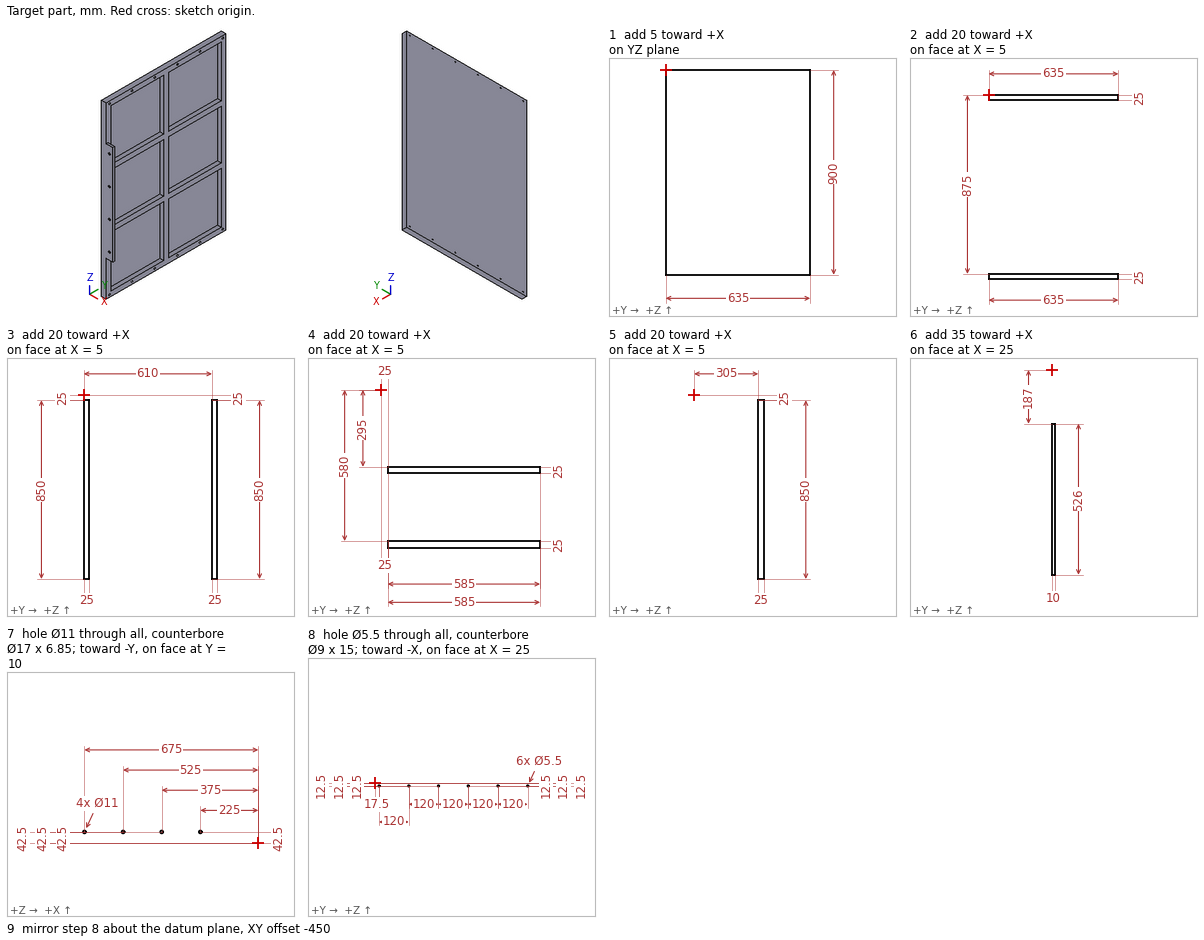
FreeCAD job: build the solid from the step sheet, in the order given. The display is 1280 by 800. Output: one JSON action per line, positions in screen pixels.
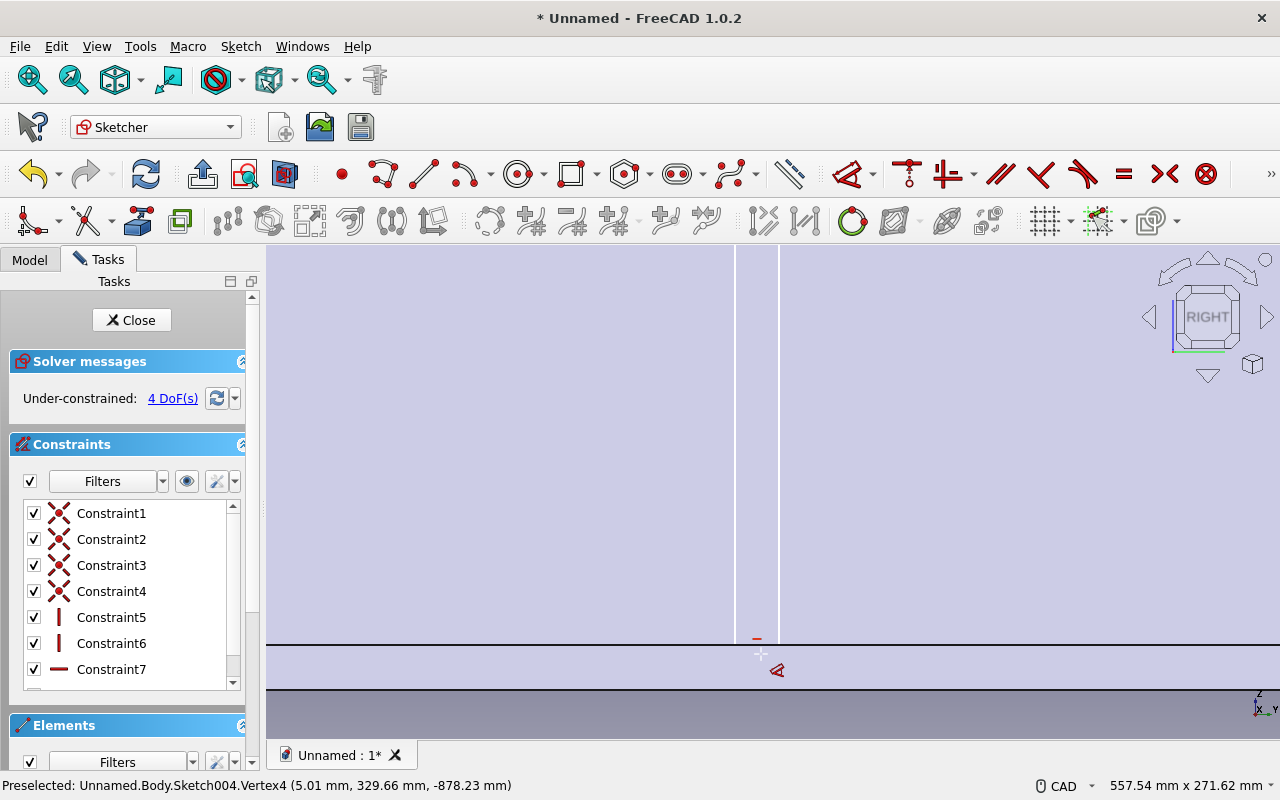
{"action": "left_click", "coordinate": [757, 651]}
{"action": "left_click", "coordinate": [757, 685]}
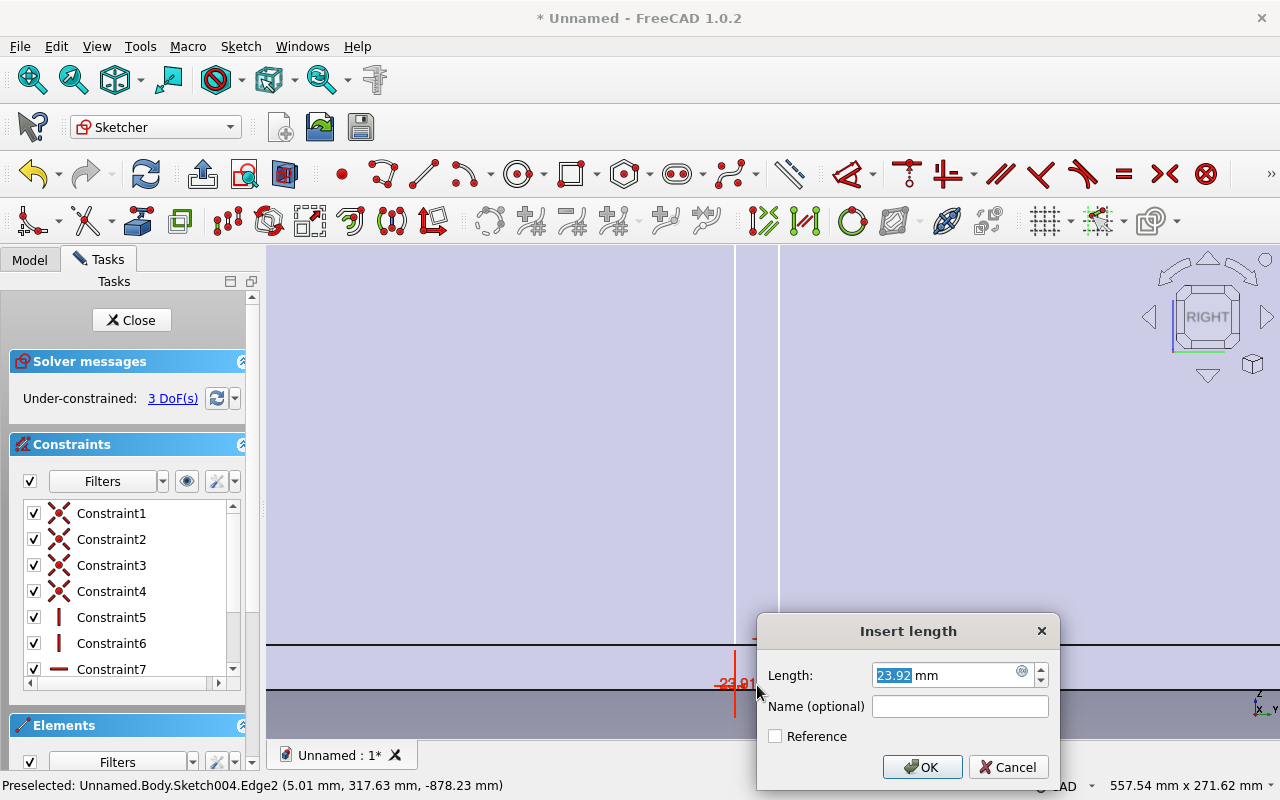
{"action": "type", "text": "25"}
{"action": "key", "text": "Return"}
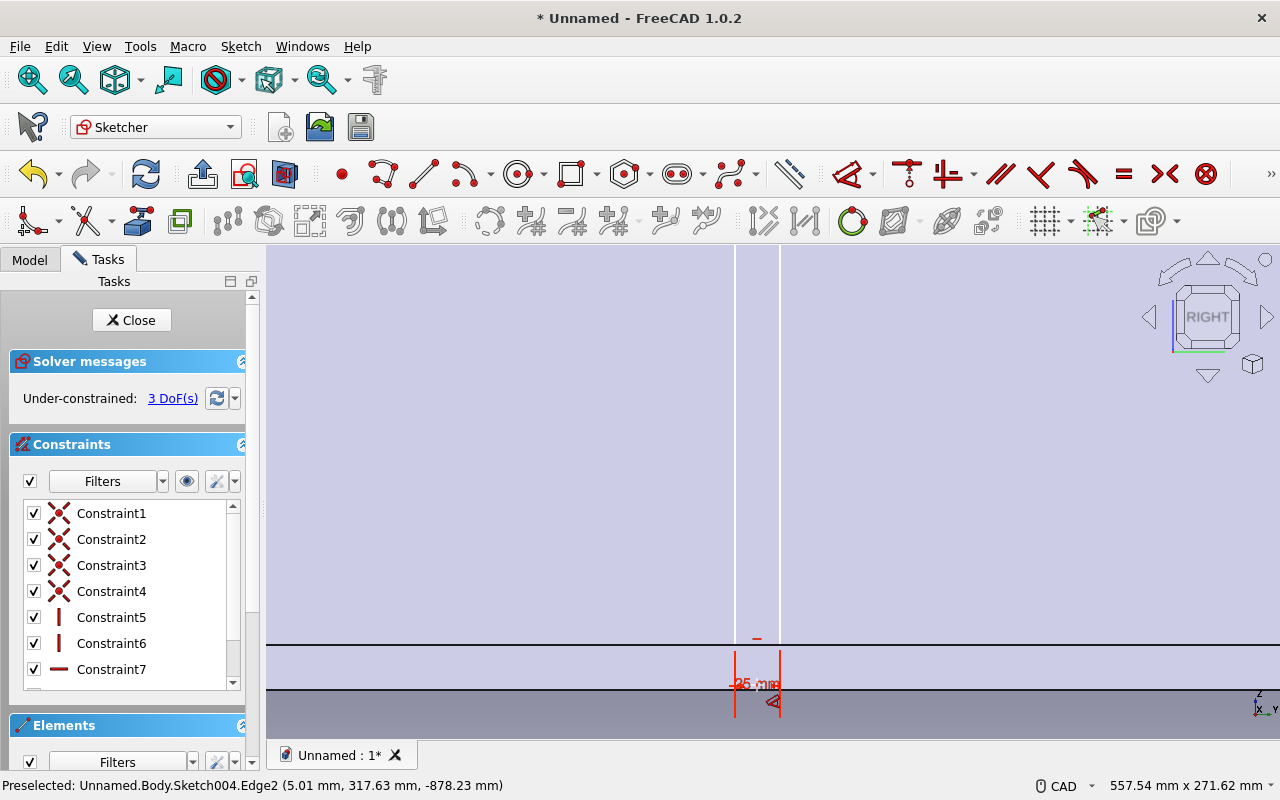
{"action": "scroll", "coordinate": [761, 655], "scroll_direction": "down", "scroll_amount": 8}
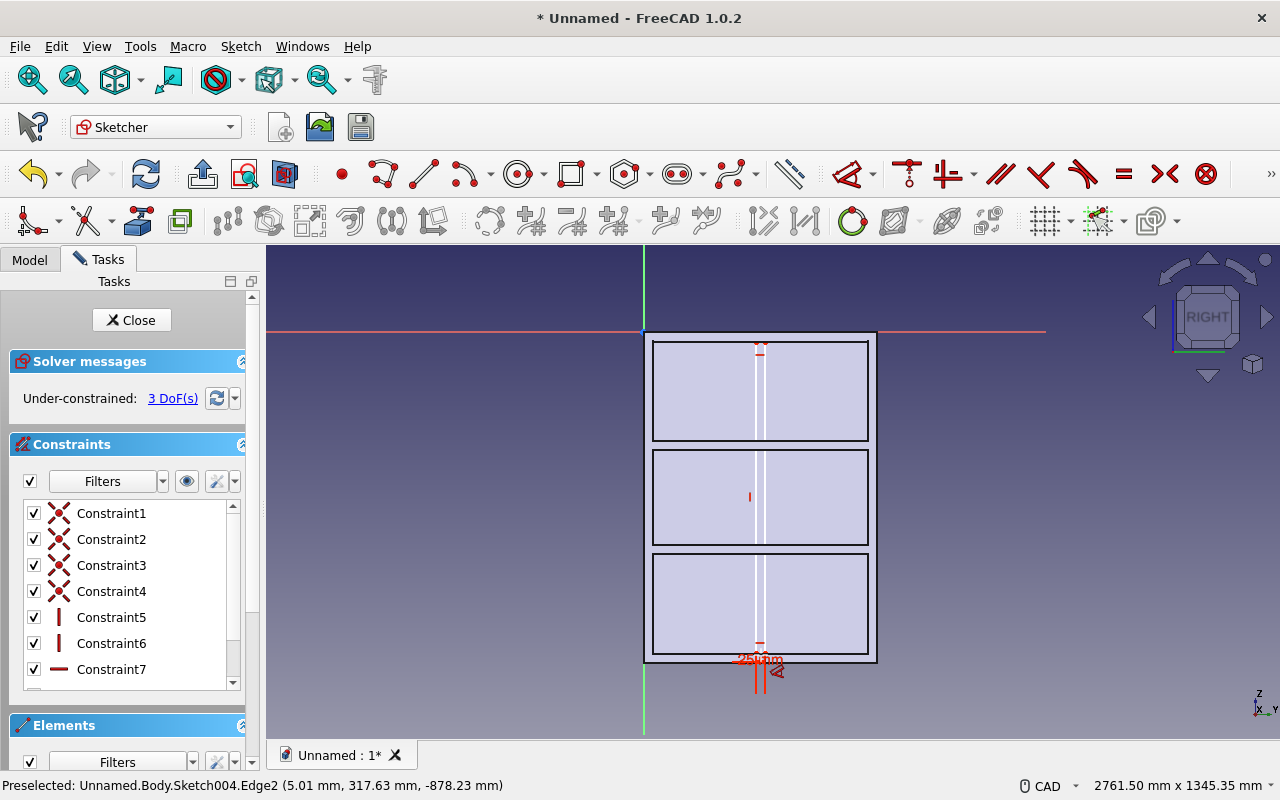
{"action": "scroll", "coordinate": [756, 592], "scroll_direction": "up", "scroll_amount": 3}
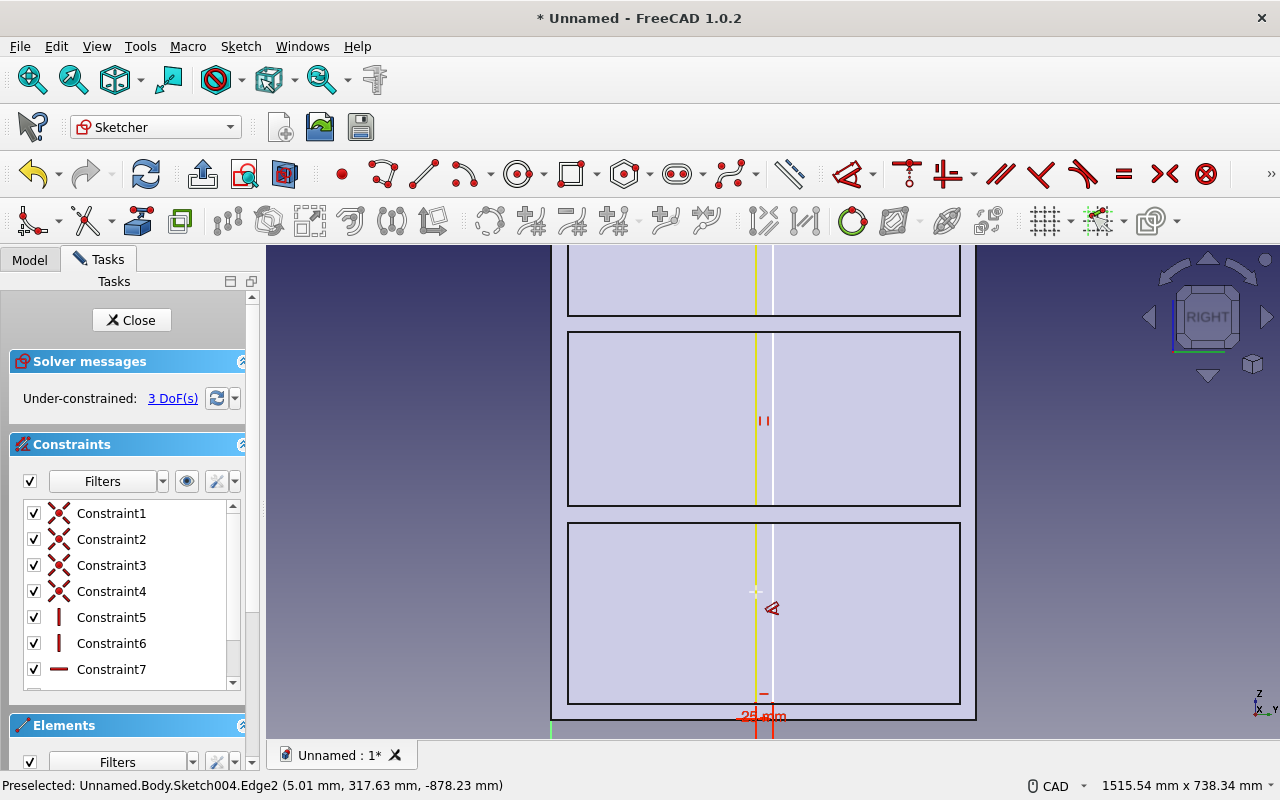
{"action": "left_click", "coordinate": [756, 592]}
{"action": "left_click", "coordinate": [790, 489]}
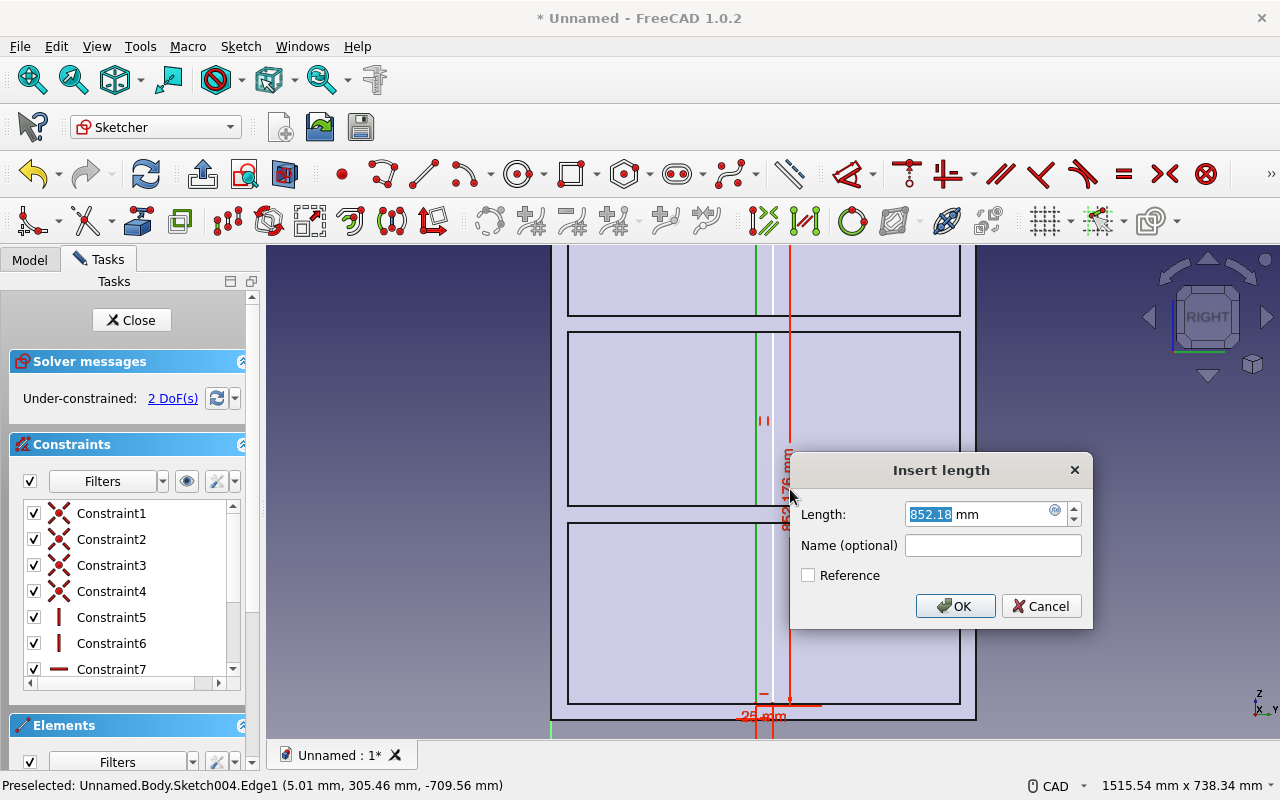
{"action": "type", "text": "850"}
{"action": "key", "text": "Return"}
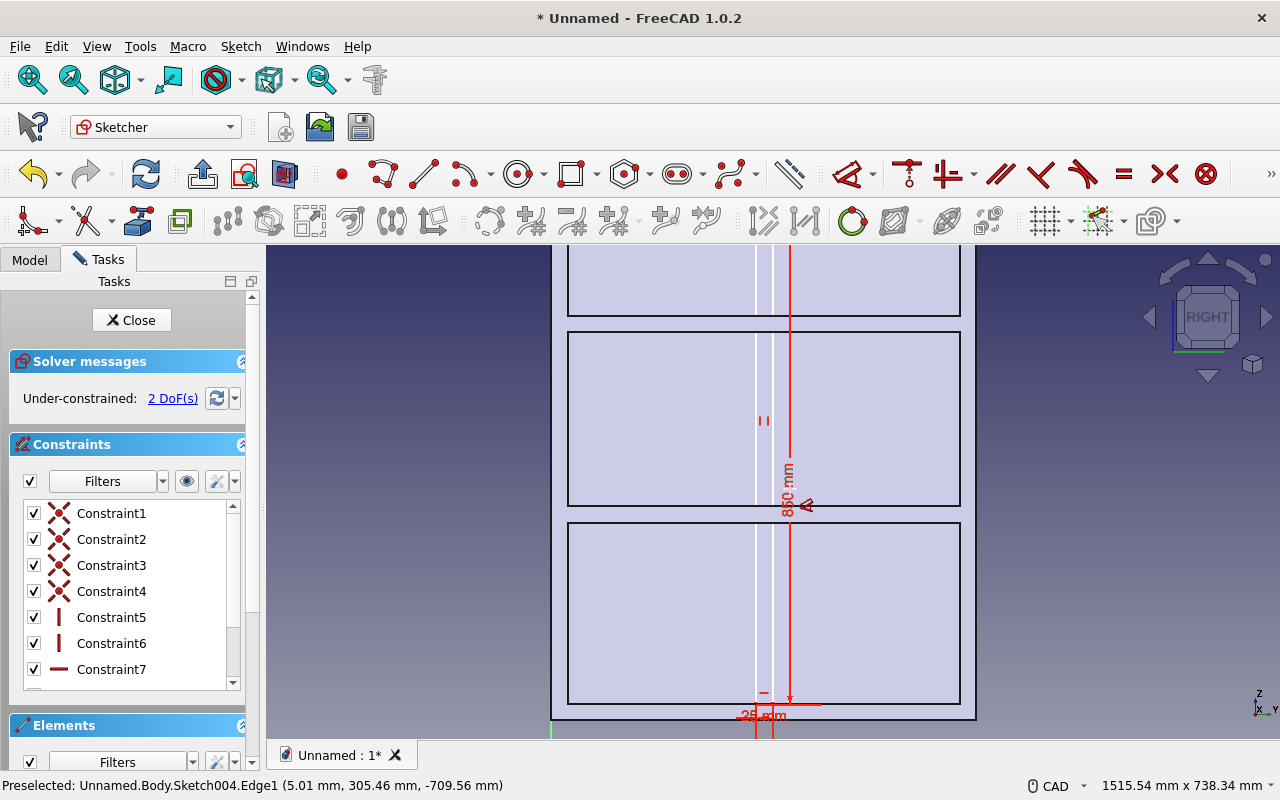
{"action": "scroll", "coordinate": [756, 591], "scroll_direction": "down", "scroll_amount": 3}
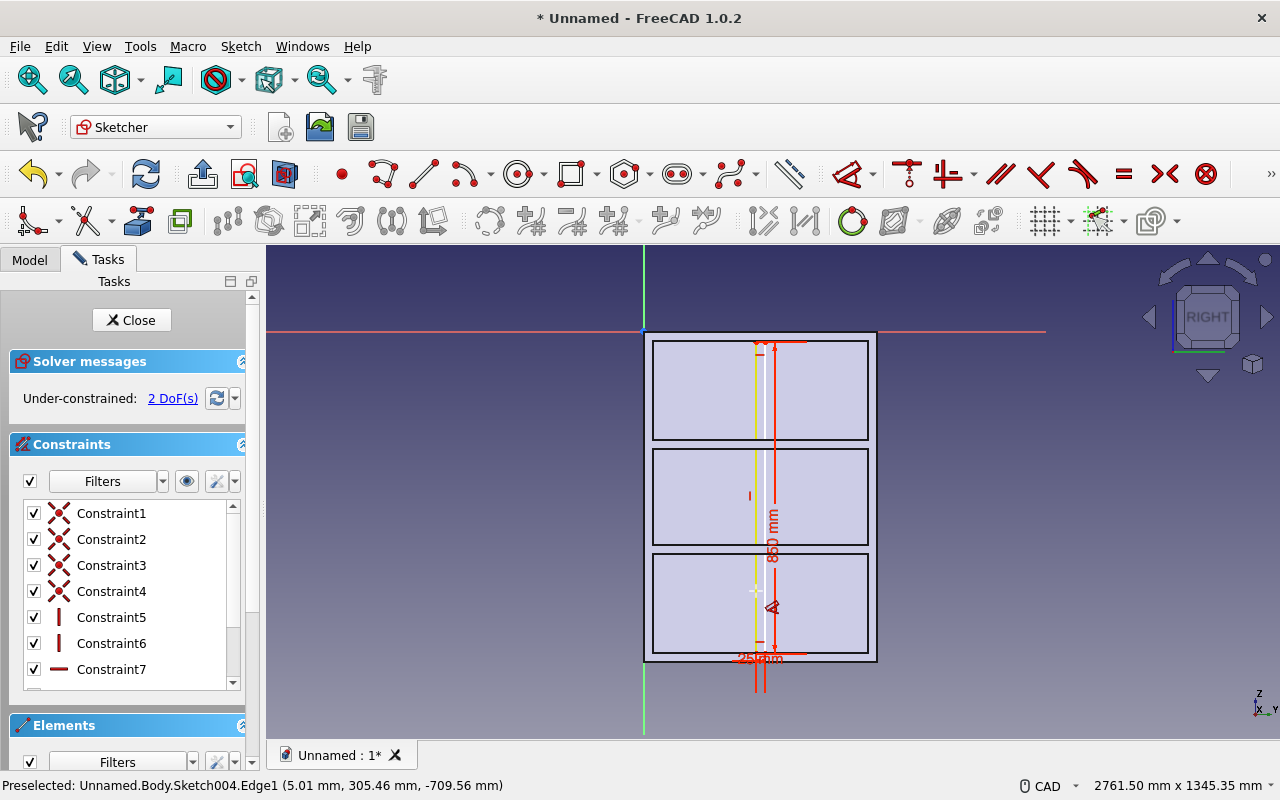
{"action": "scroll", "coordinate": [756, 342], "scroll_direction": "up", "scroll_amount": 8}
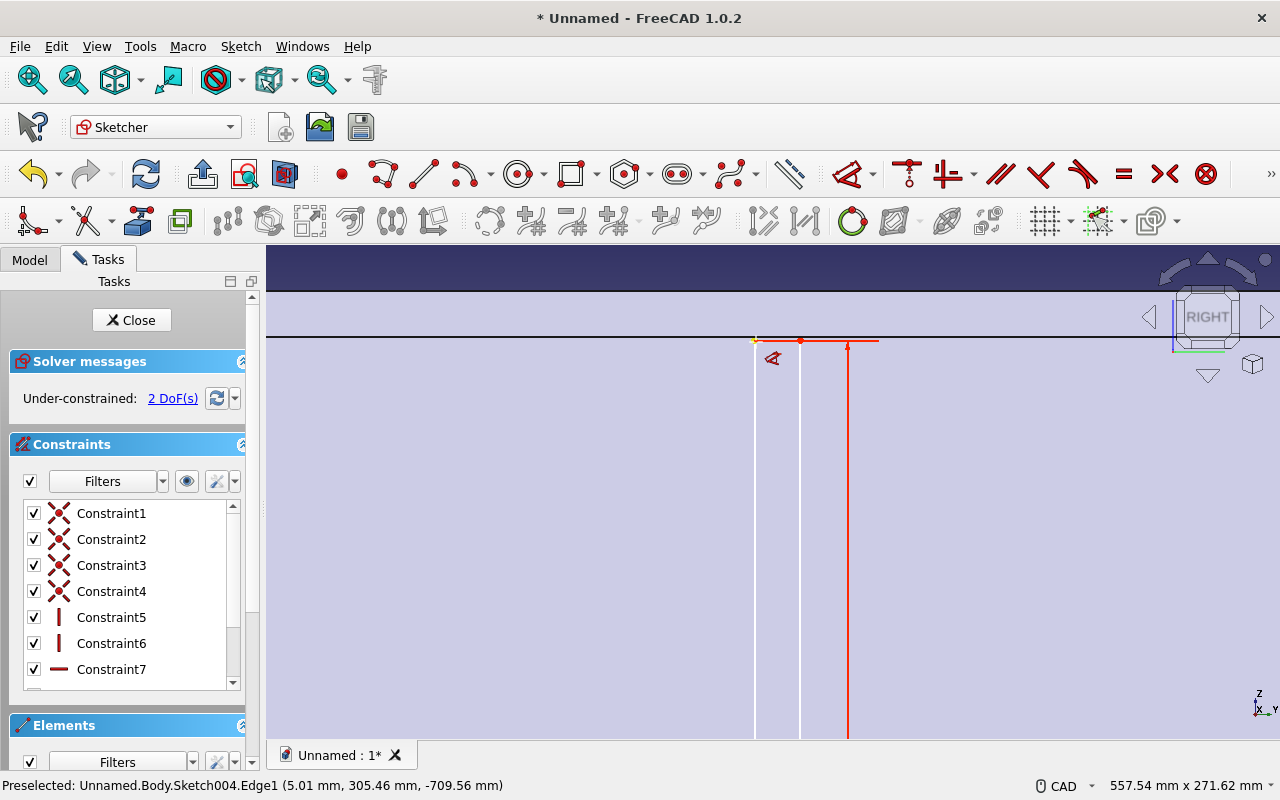
{"action": "left_click", "coordinate": [755, 341]}
{"action": "left_click", "coordinate": [789, 316]}